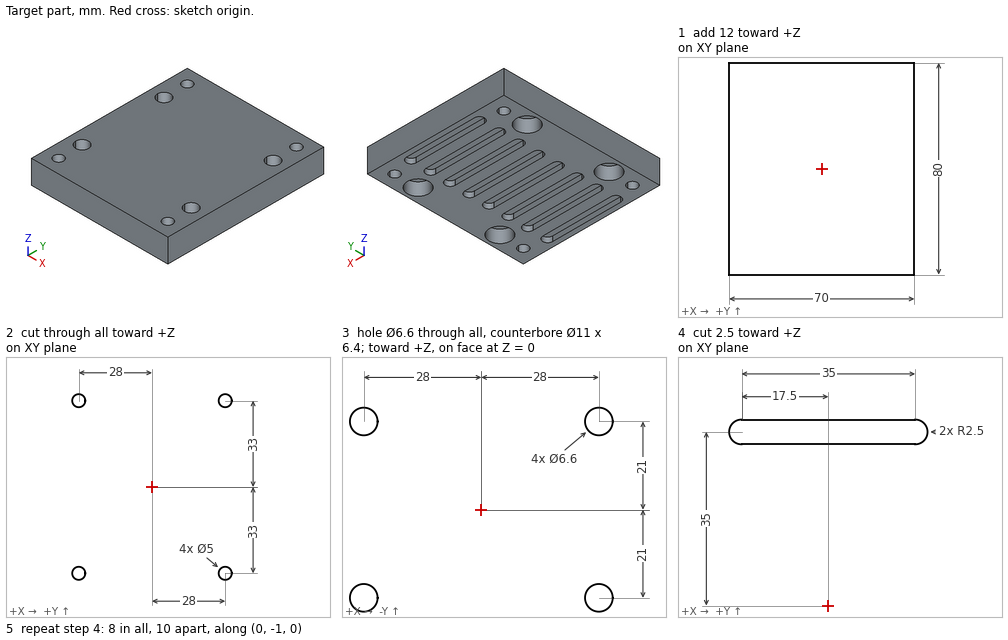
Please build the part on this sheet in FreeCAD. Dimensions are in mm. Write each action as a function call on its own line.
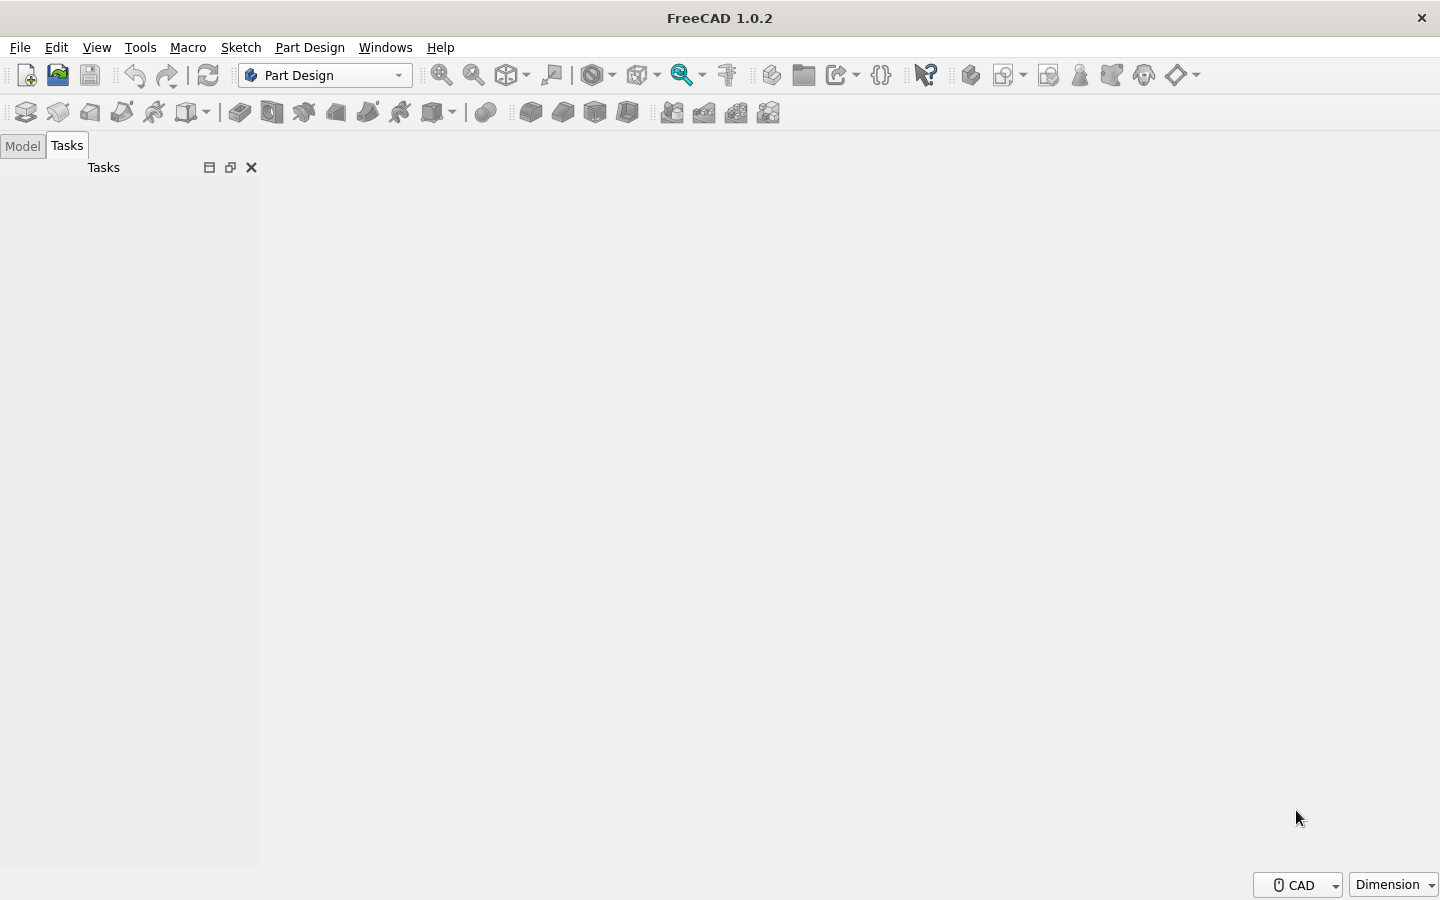
key(ctrl+n)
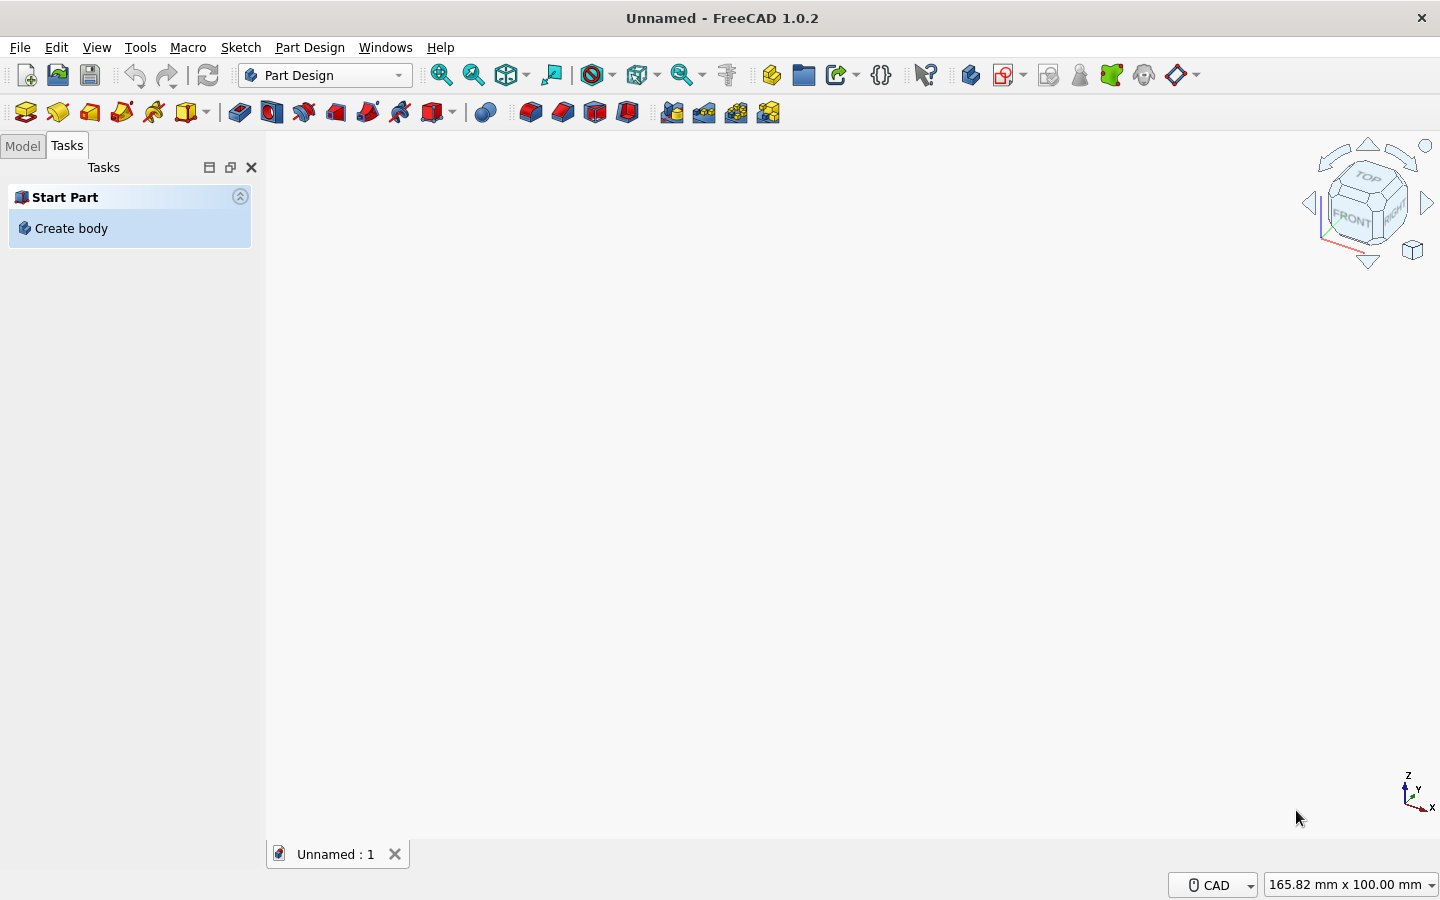
click(1004, 76)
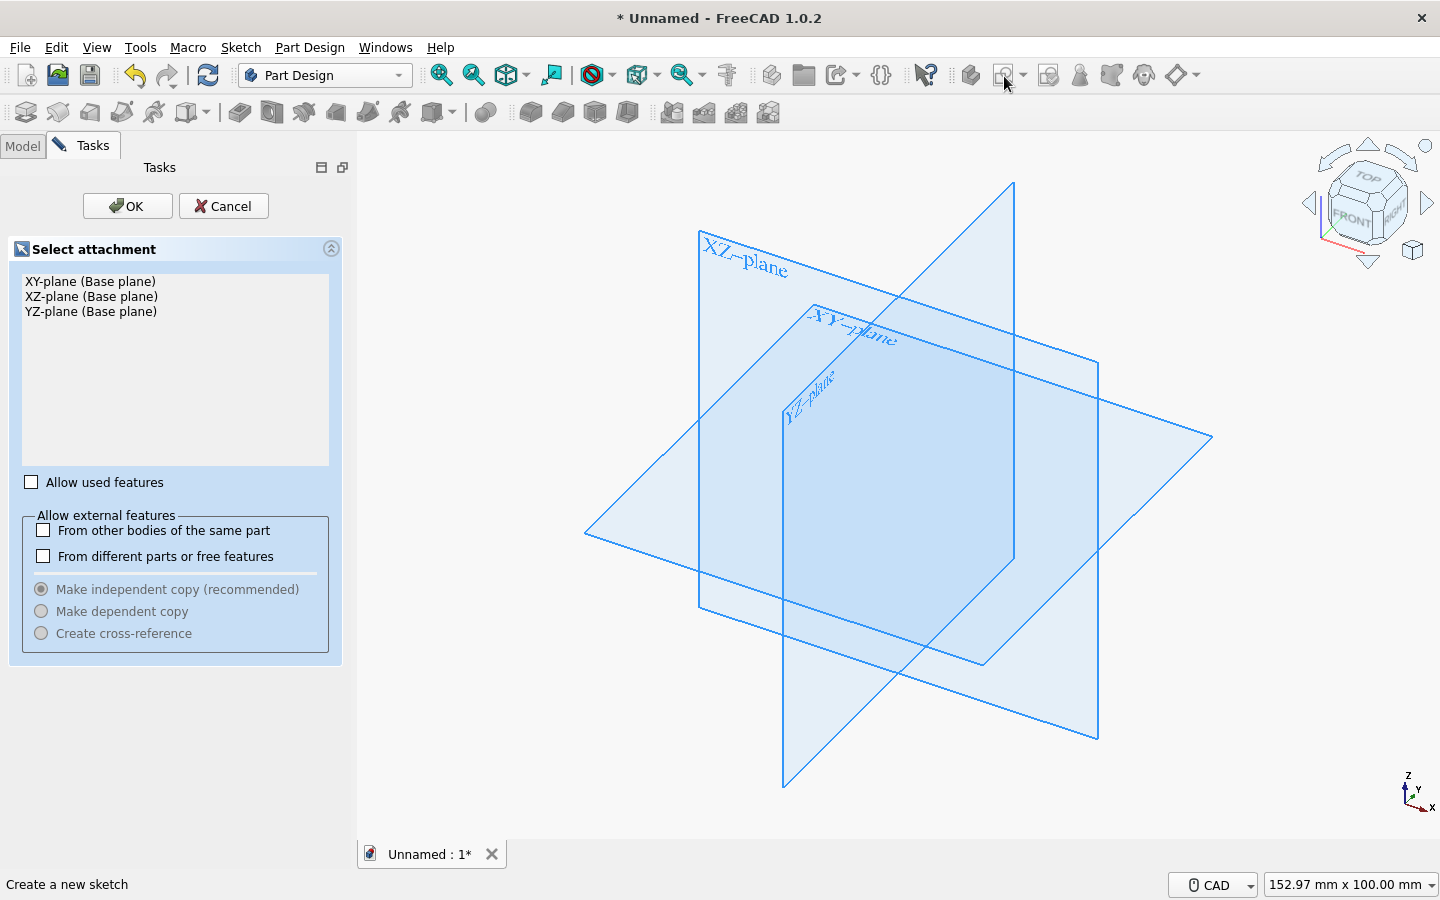
click(82, 282)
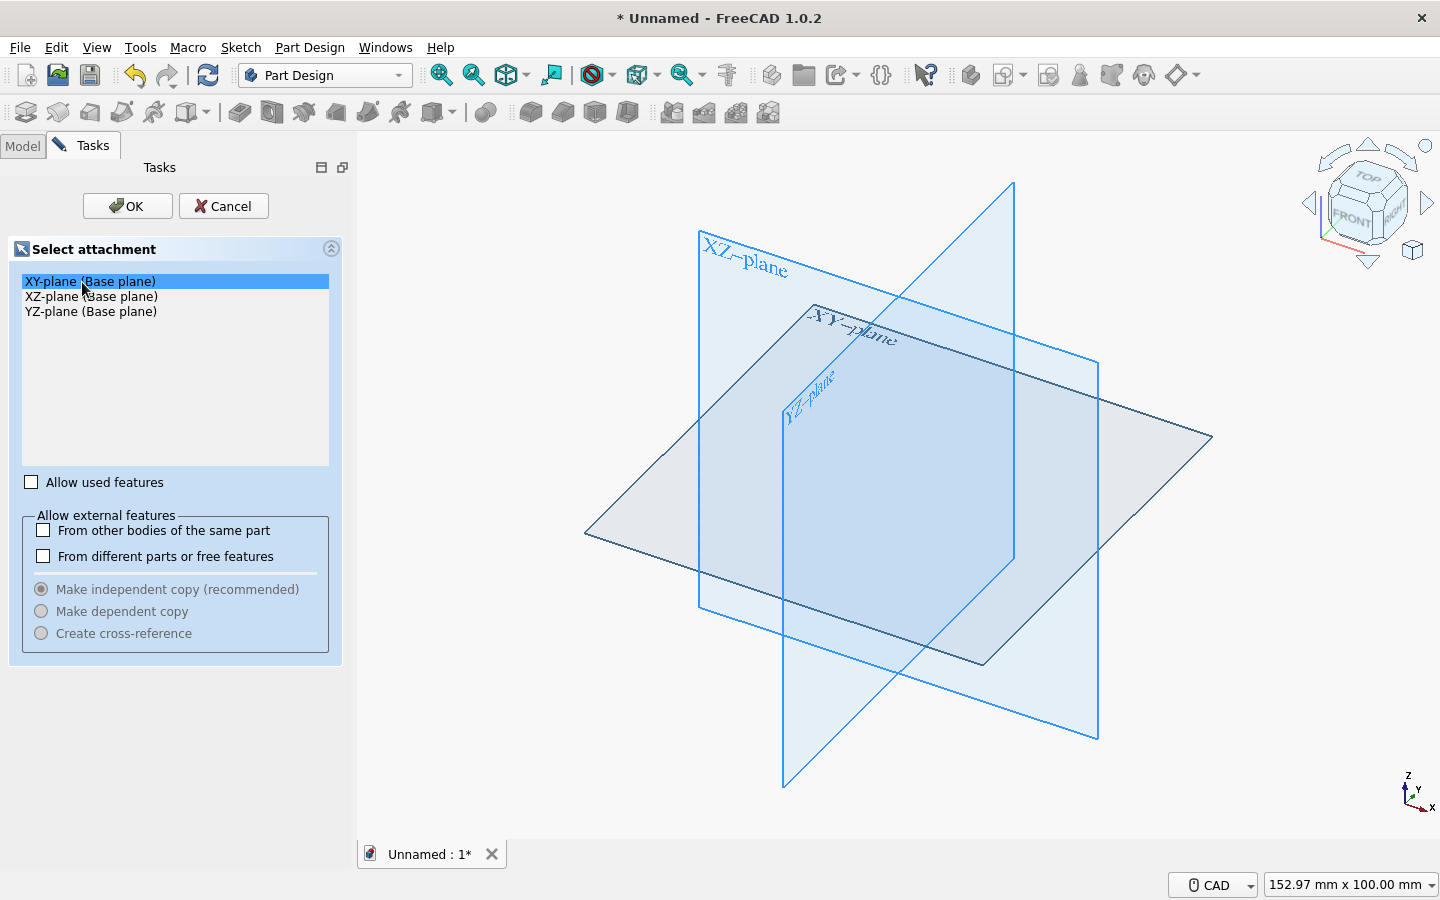
click(128, 206)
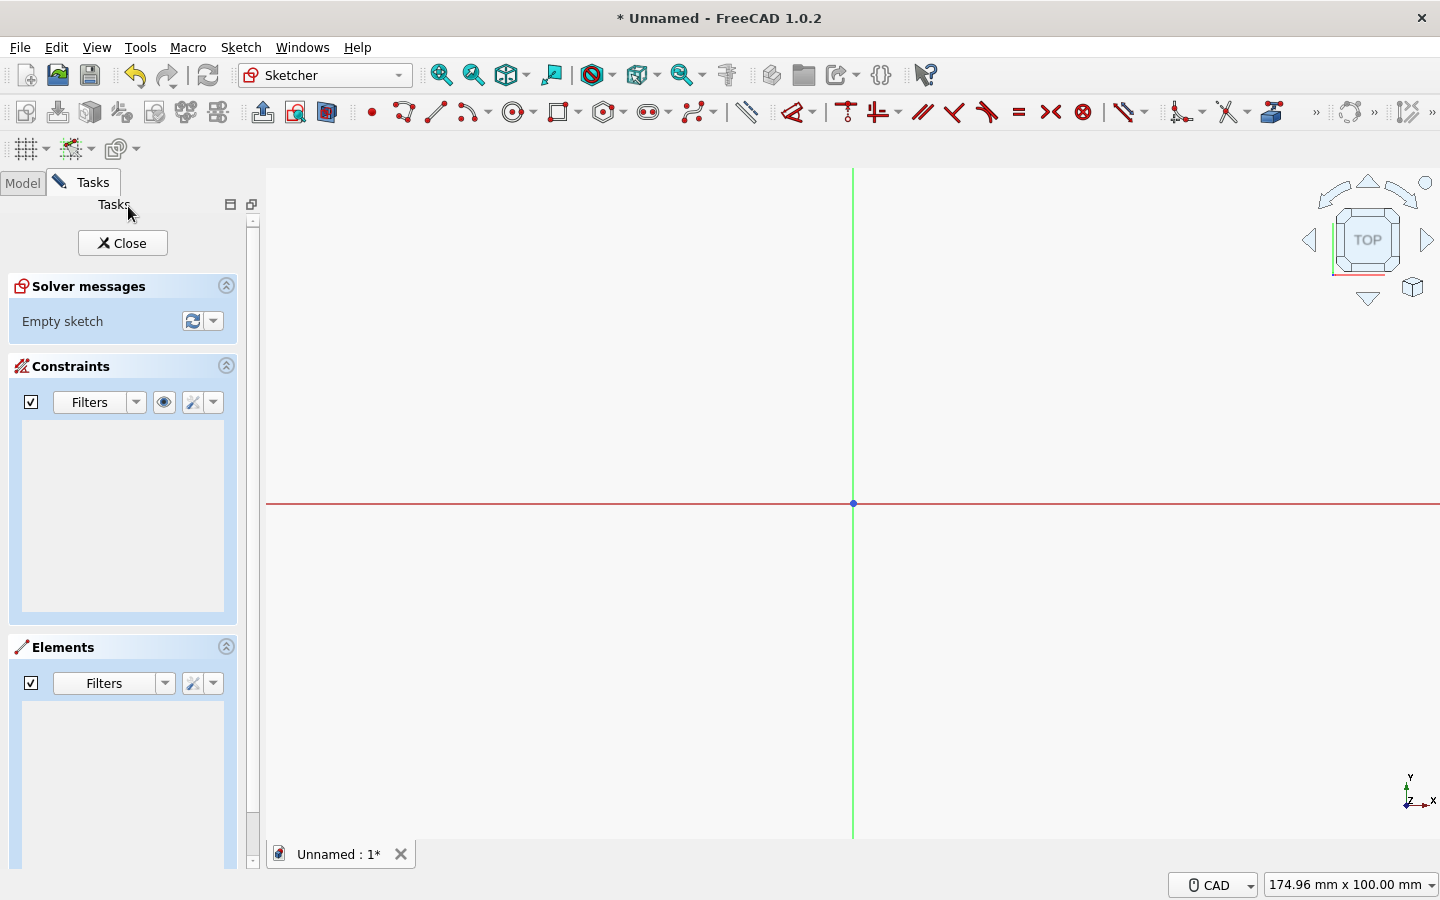
key(g)
key(v)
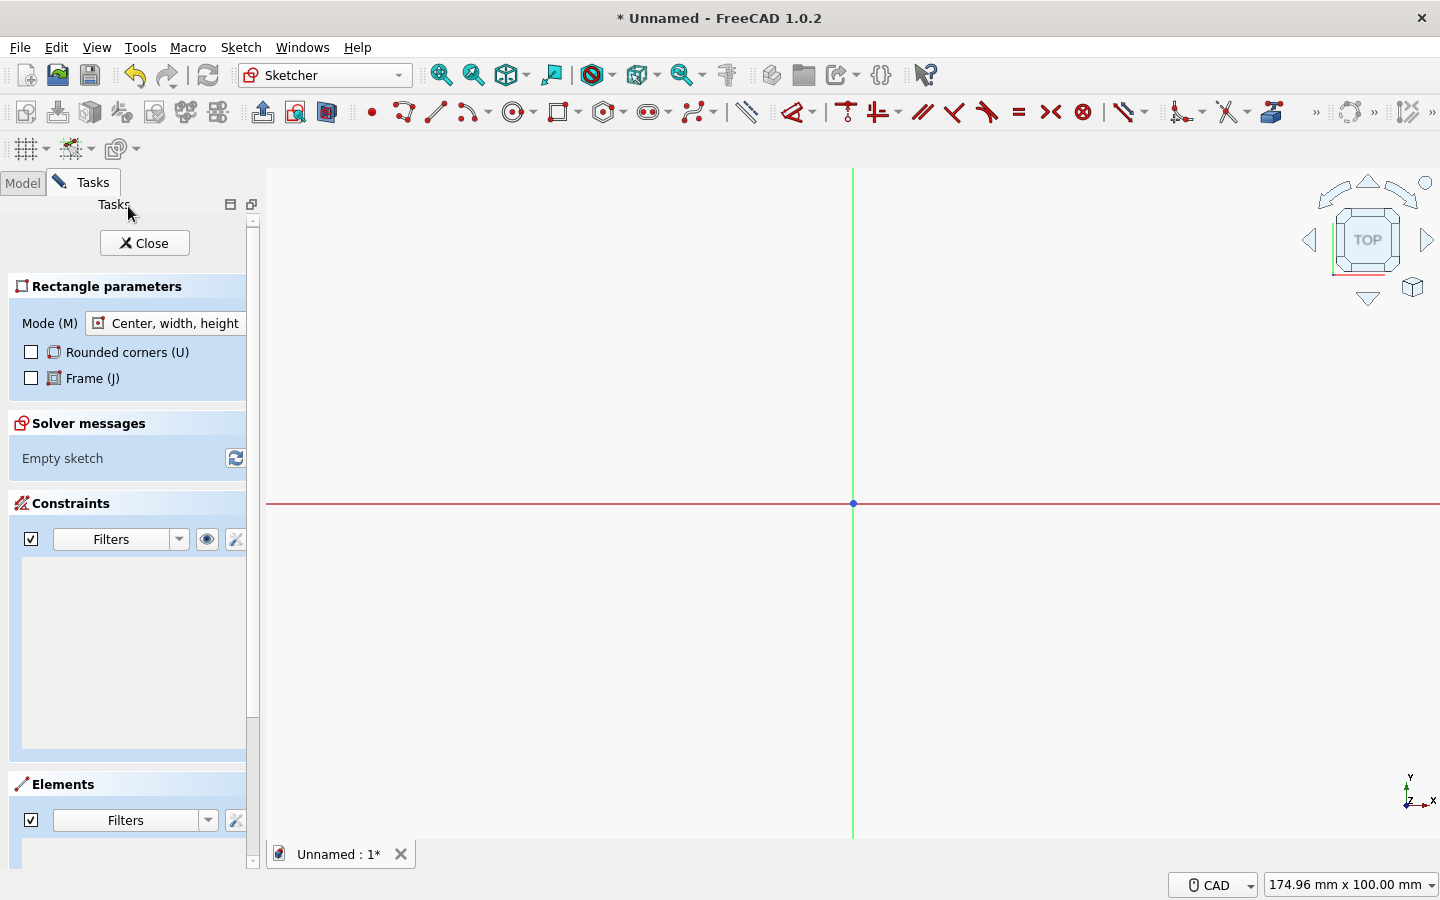
click(853, 504)
move(1088, 235)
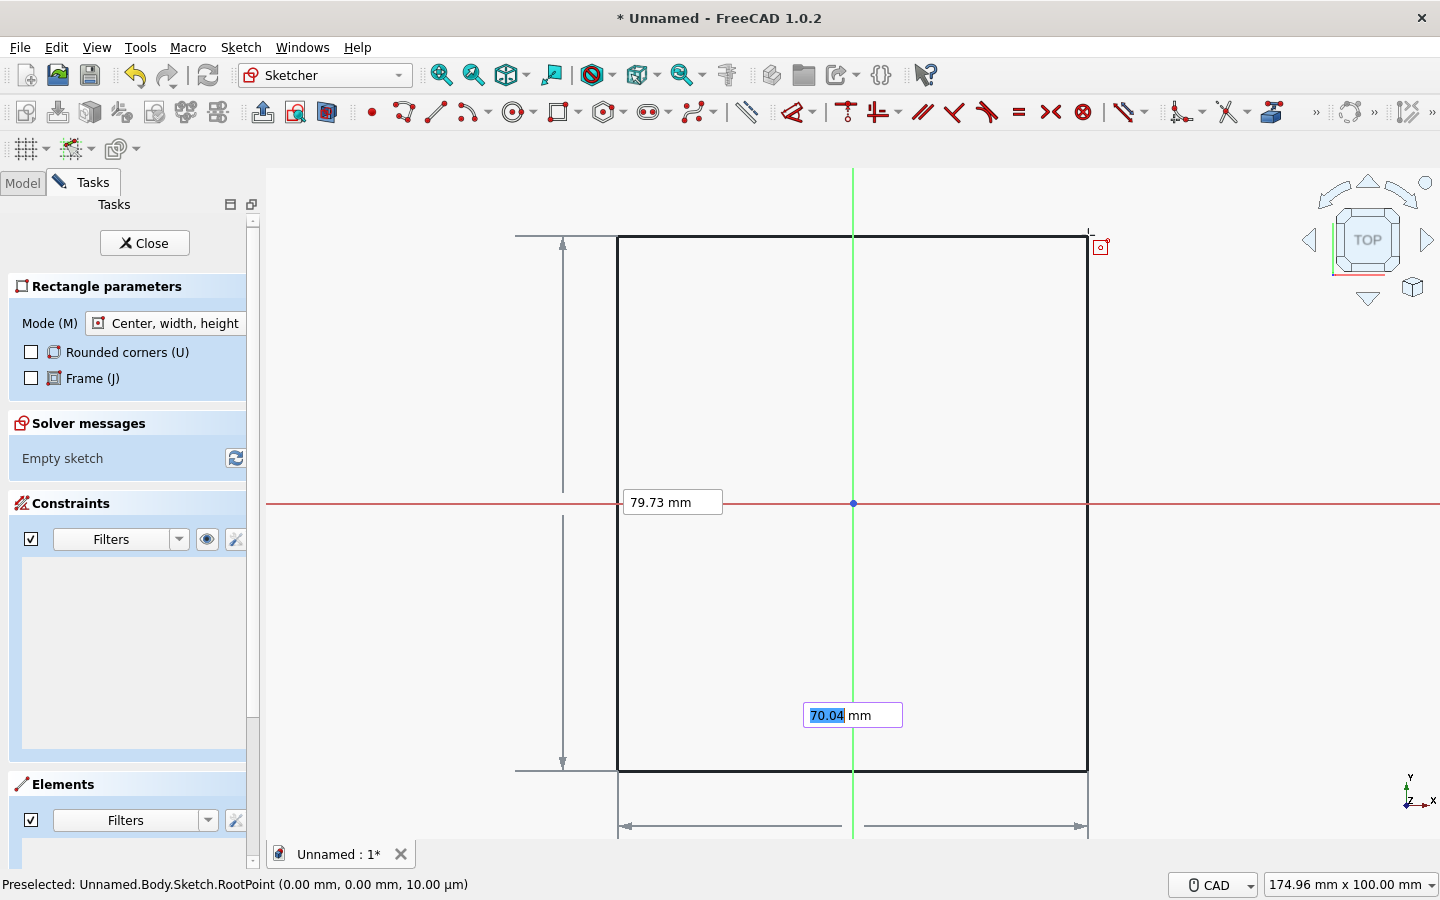
text(70)
key(Tab)
text(80)
key(Return)
key(Escape)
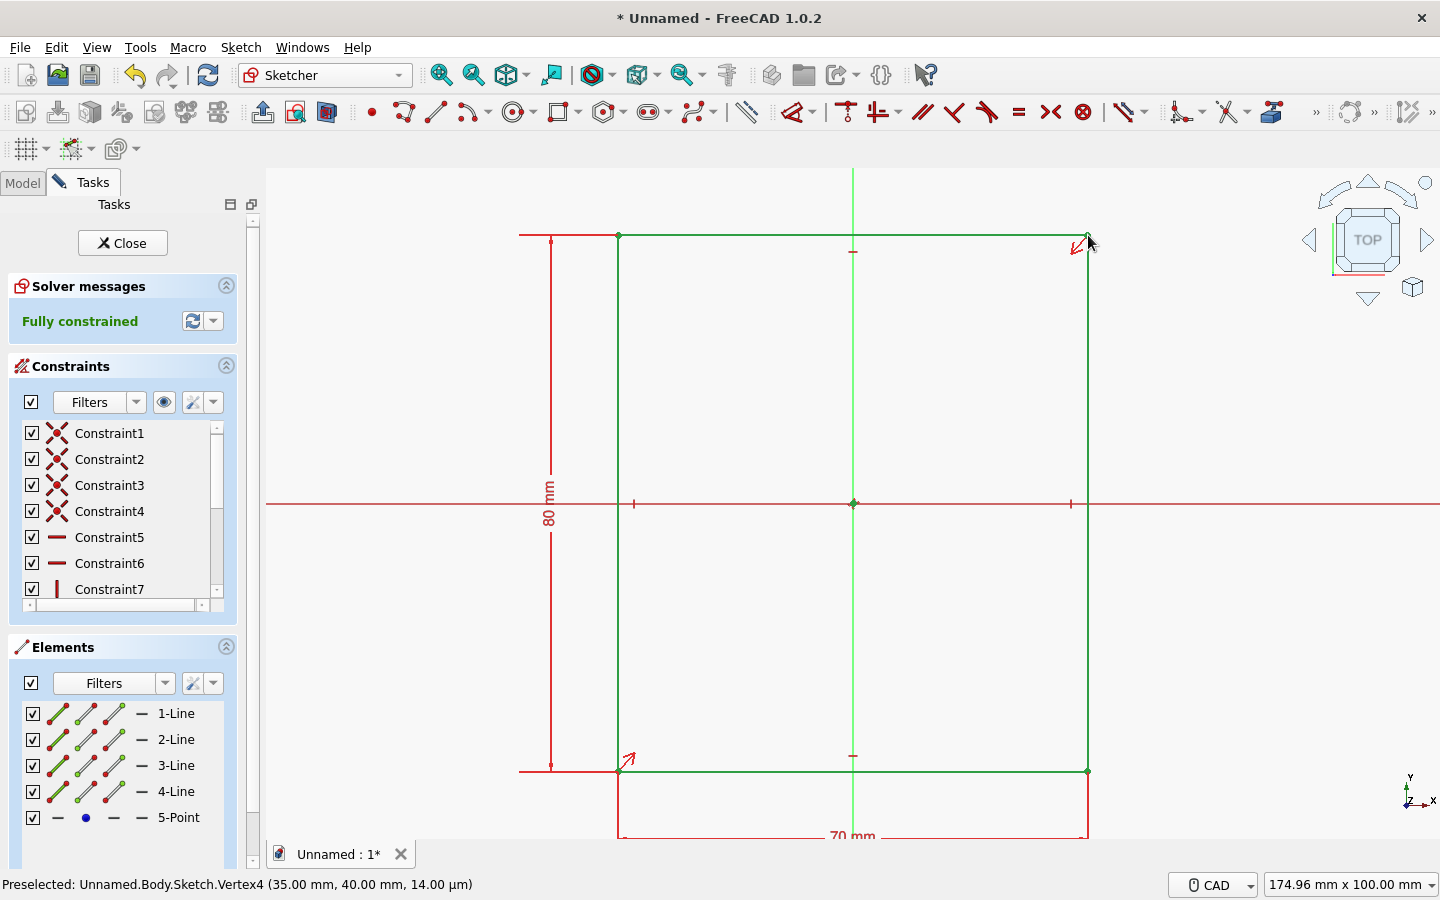
click(123, 243)